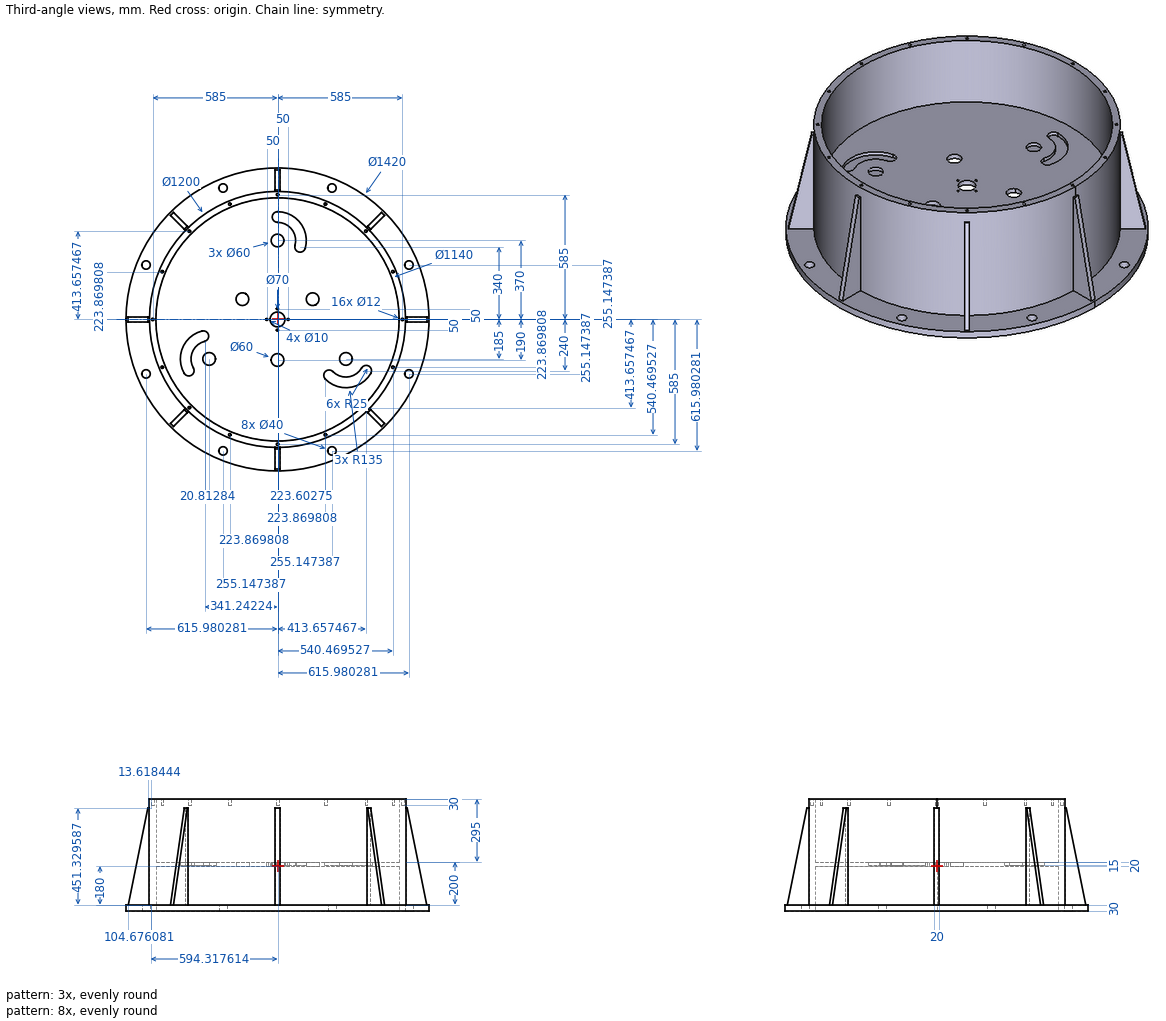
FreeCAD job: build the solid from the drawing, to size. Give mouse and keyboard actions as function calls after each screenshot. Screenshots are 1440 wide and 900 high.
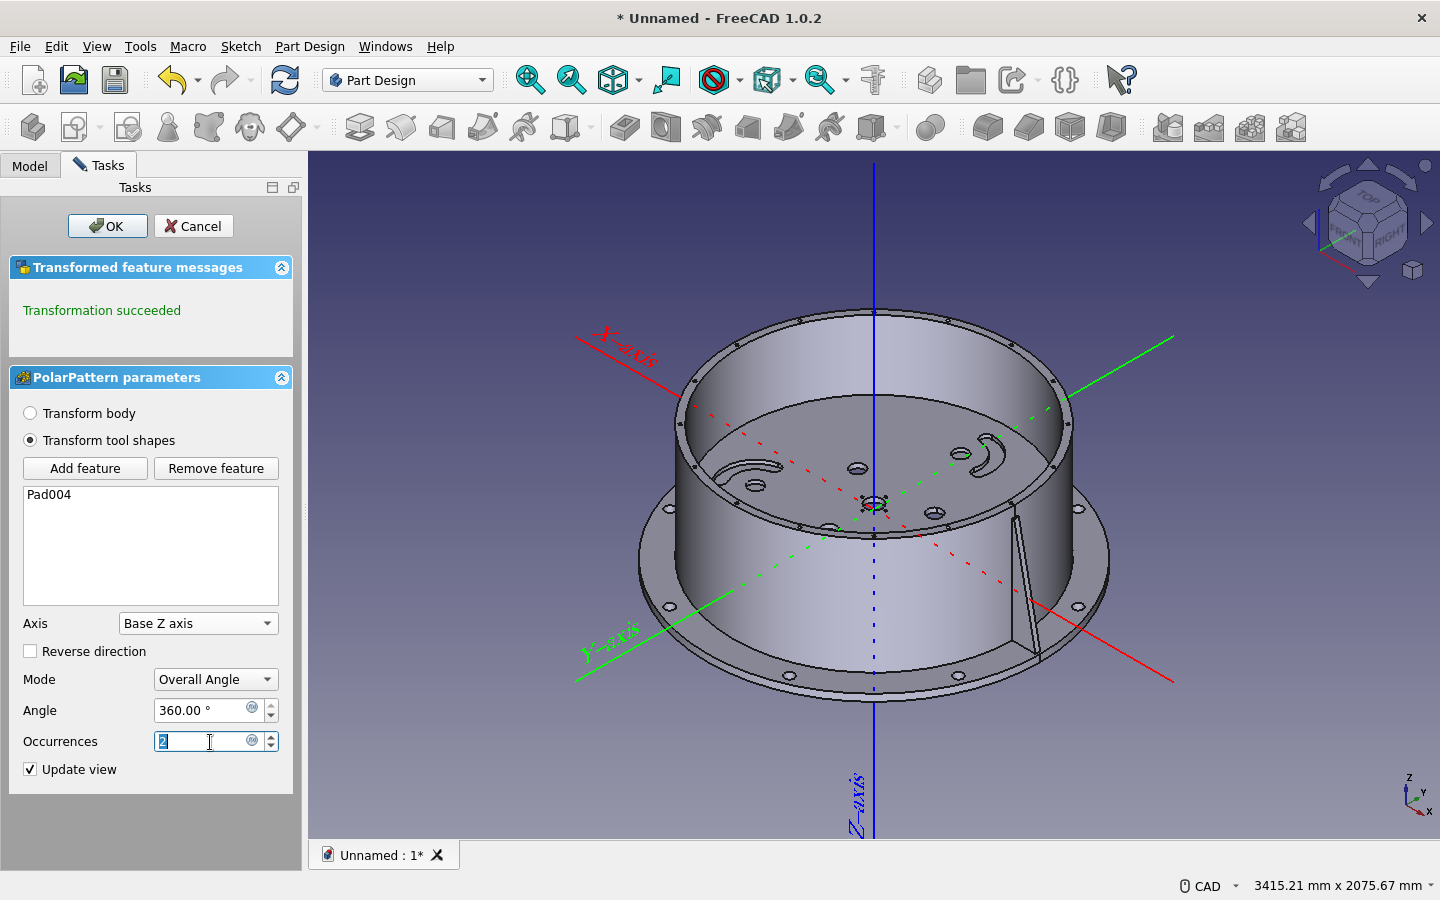
text(8)
key(Tab)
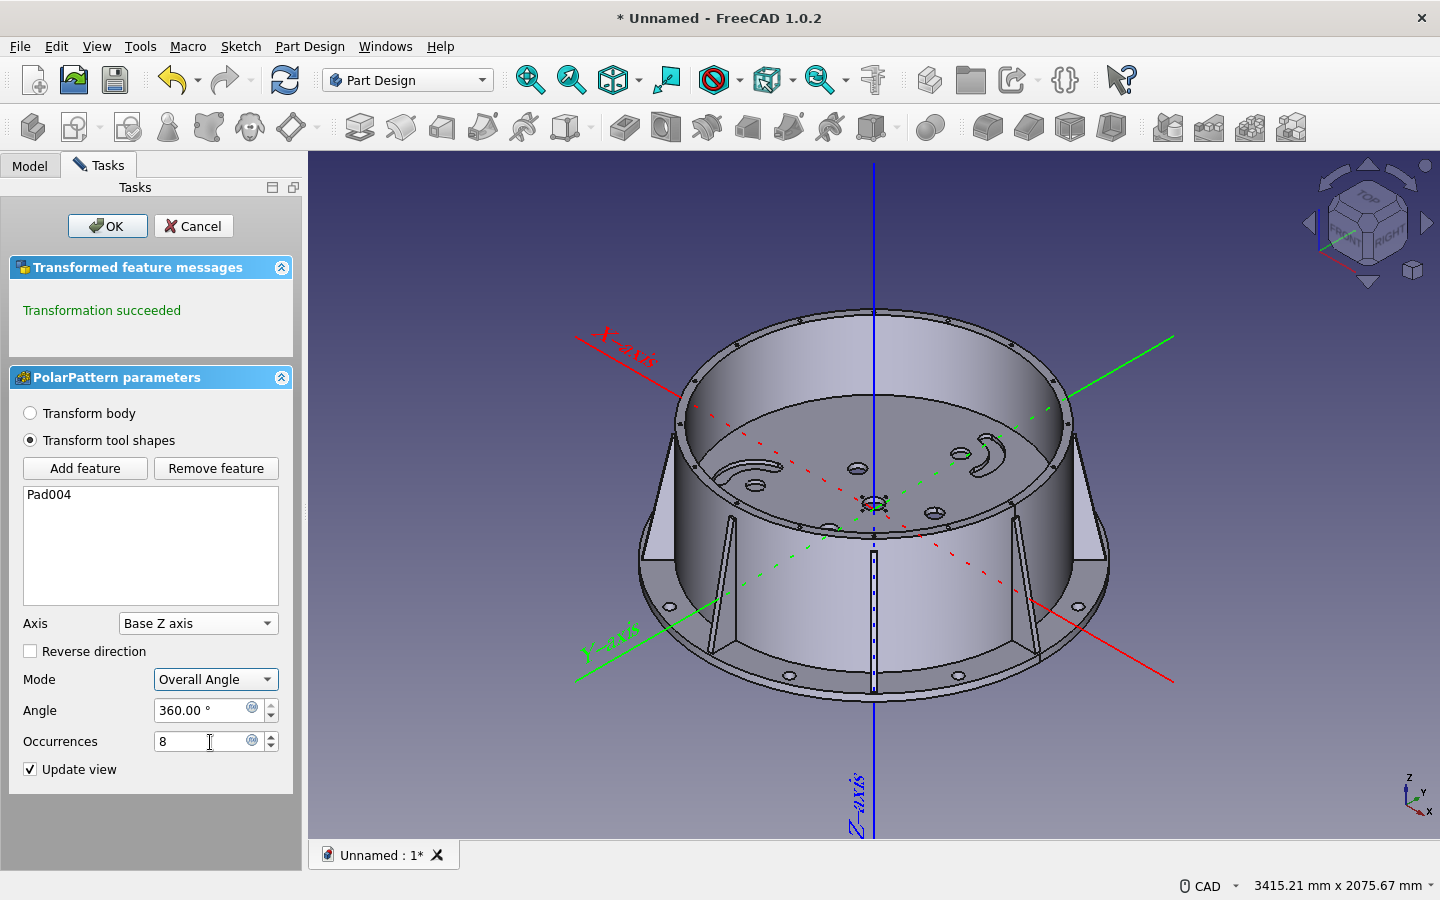
click(108, 226)